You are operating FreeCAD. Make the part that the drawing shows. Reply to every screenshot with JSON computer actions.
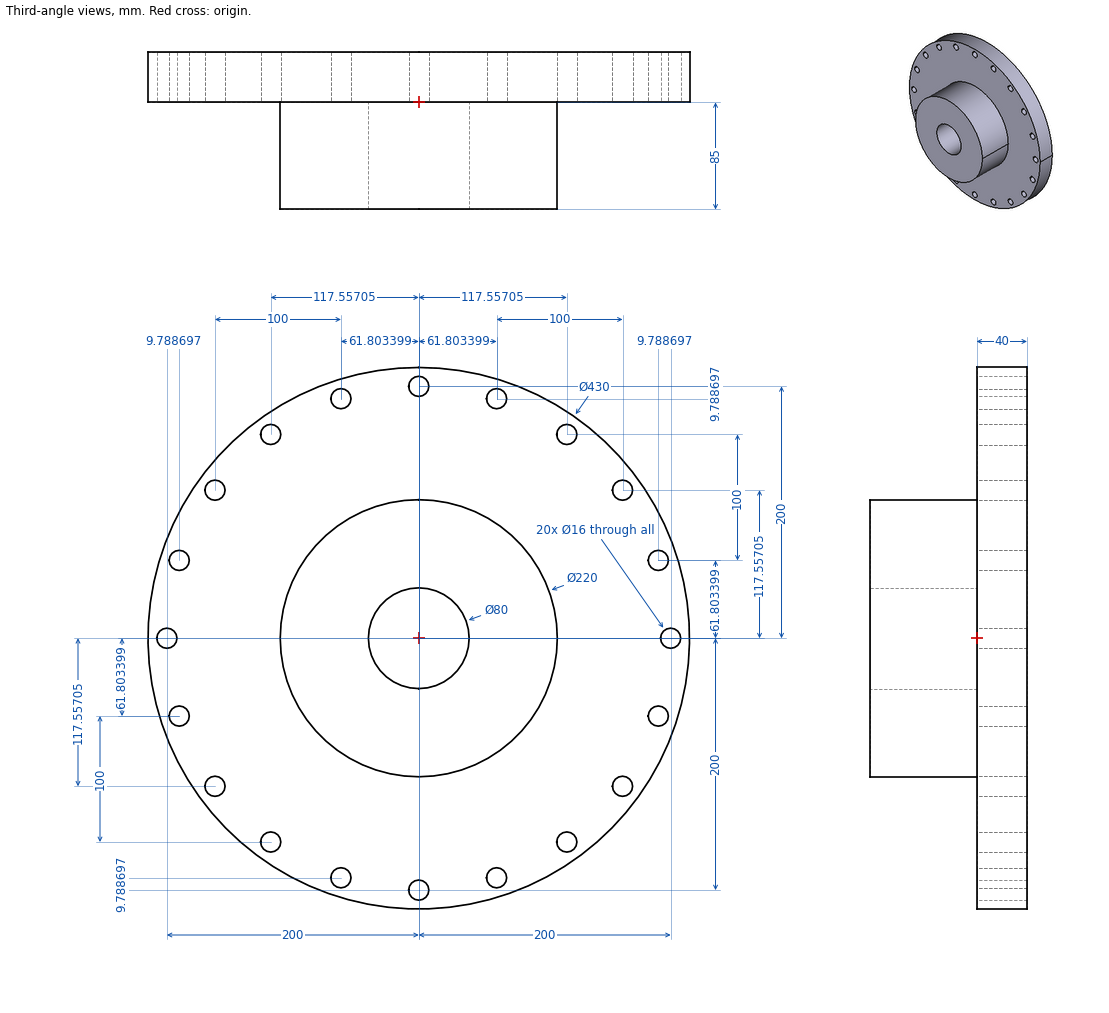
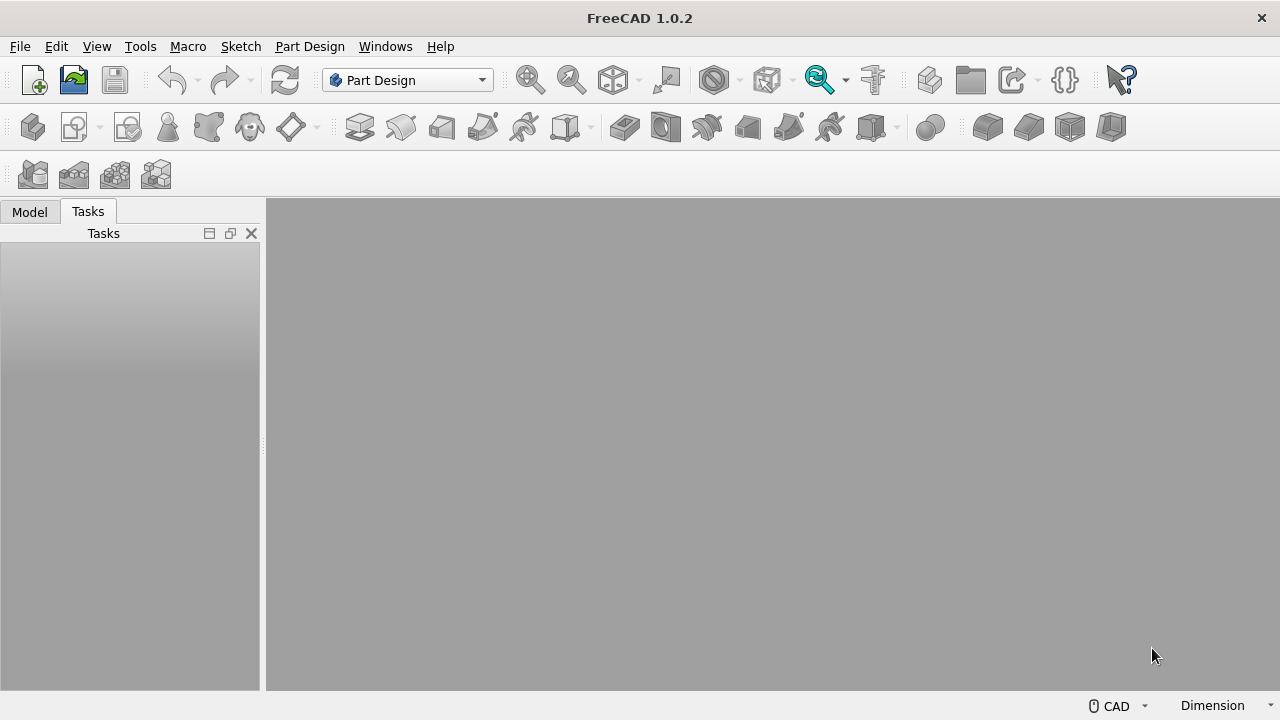
{"action": "key", "text": "ctrl+n"}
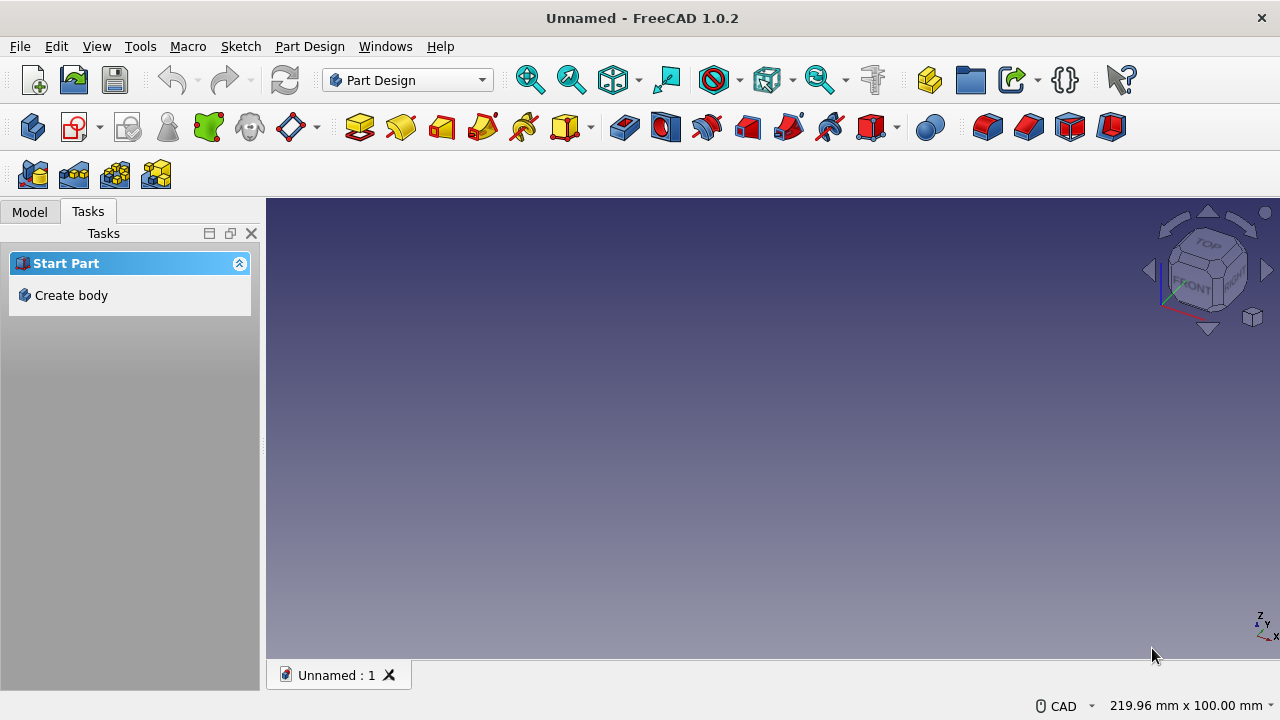
{"action": "left_click", "coordinate": [74, 128]}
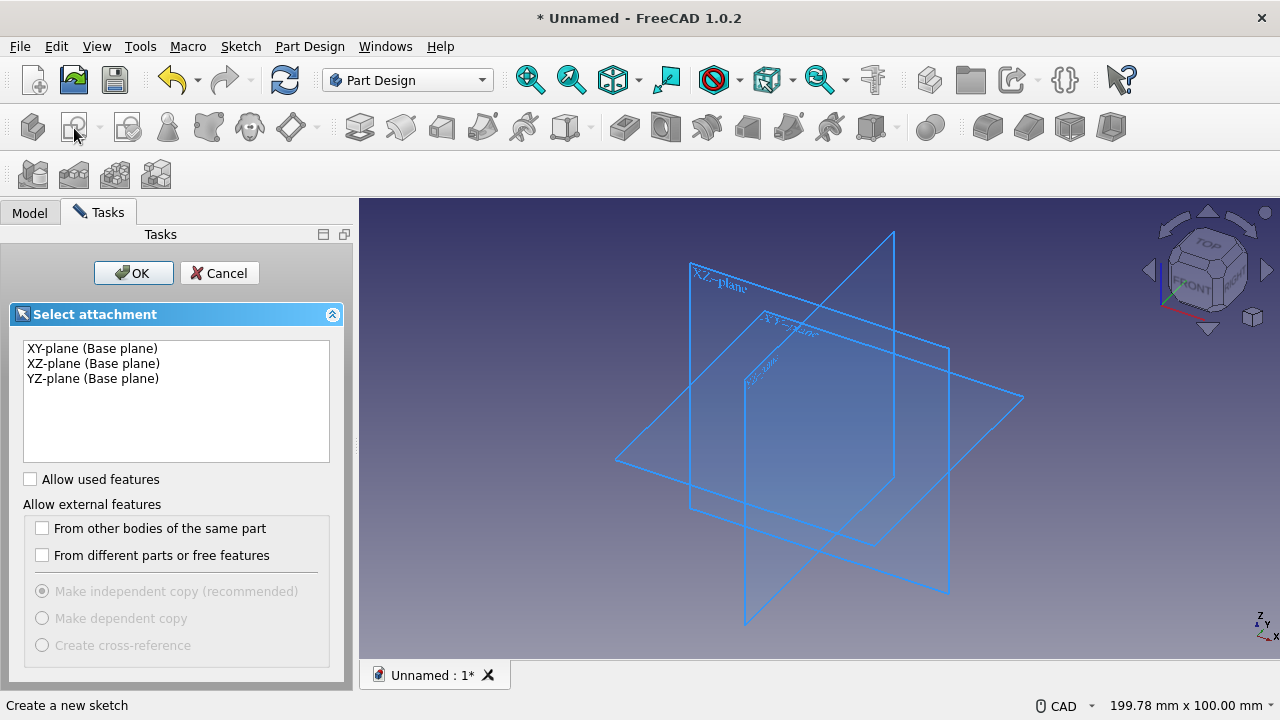
{"action": "left_click", "coordinate": [84, 364]}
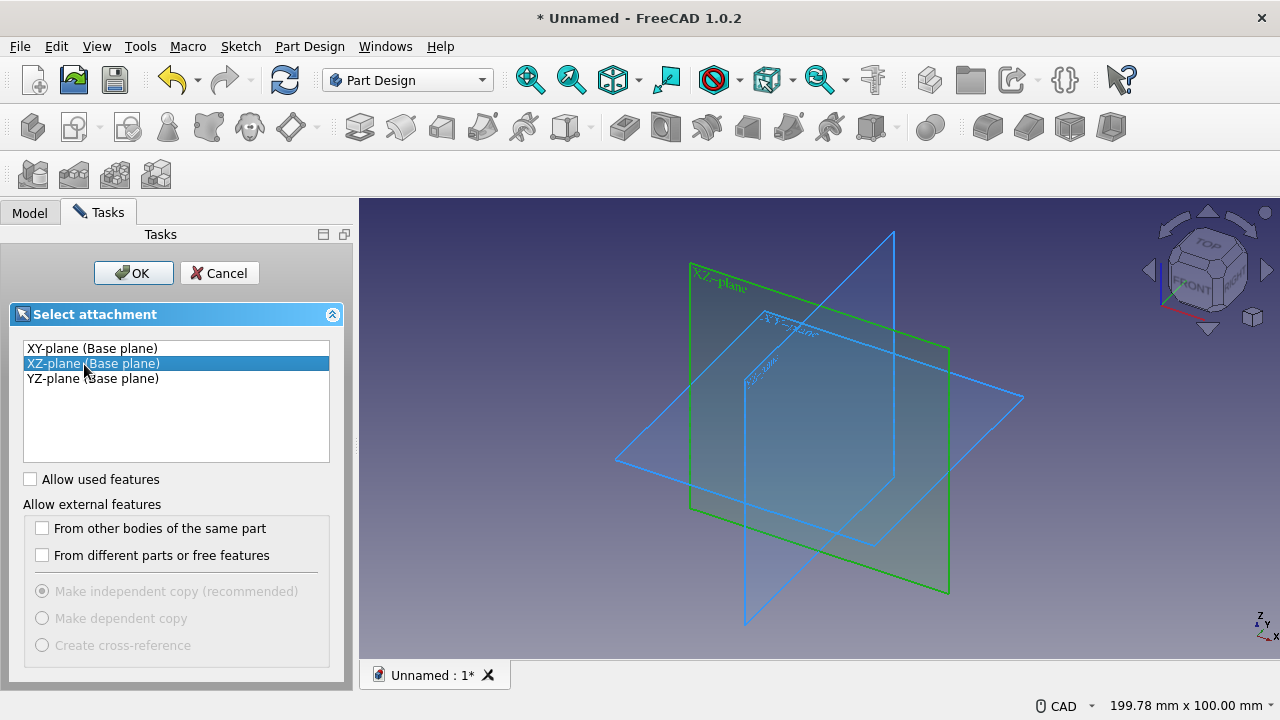
{"action": "left_click", "coordinate": [134, 273]}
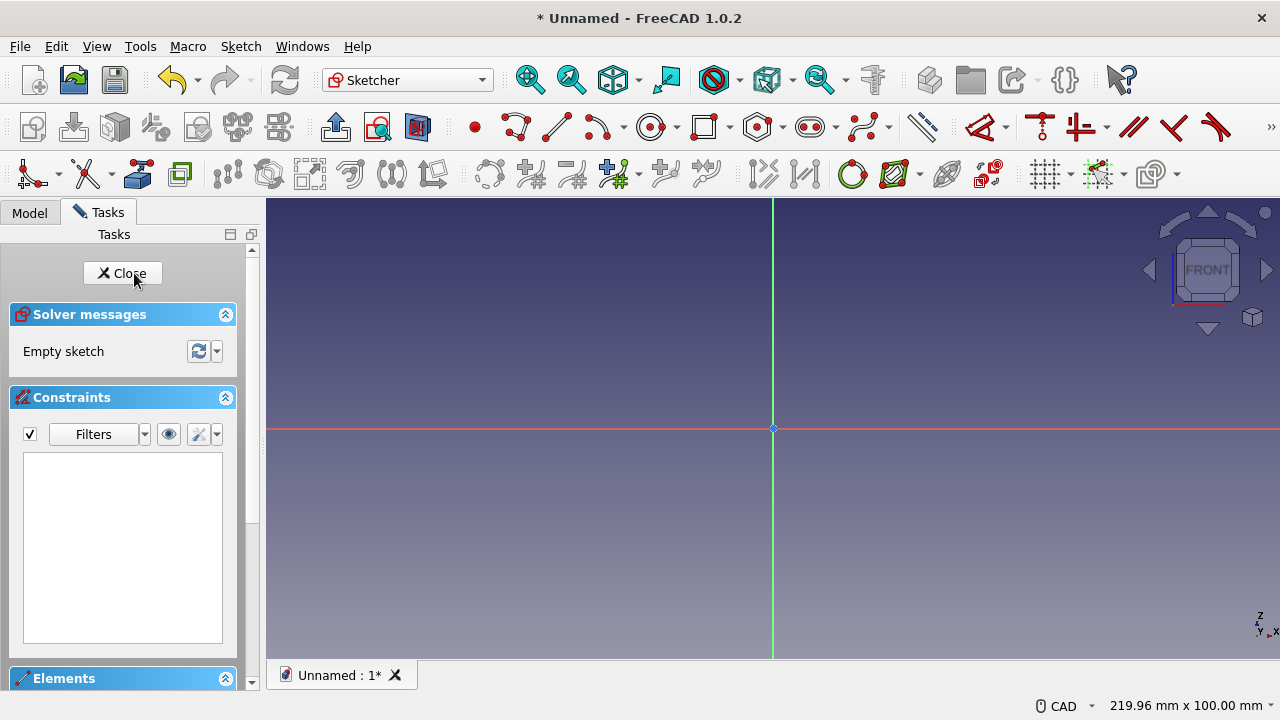
{"action": "scroll", "coordinate": [694, 428], "scroll_direction": "down", "scroll_amount": 10}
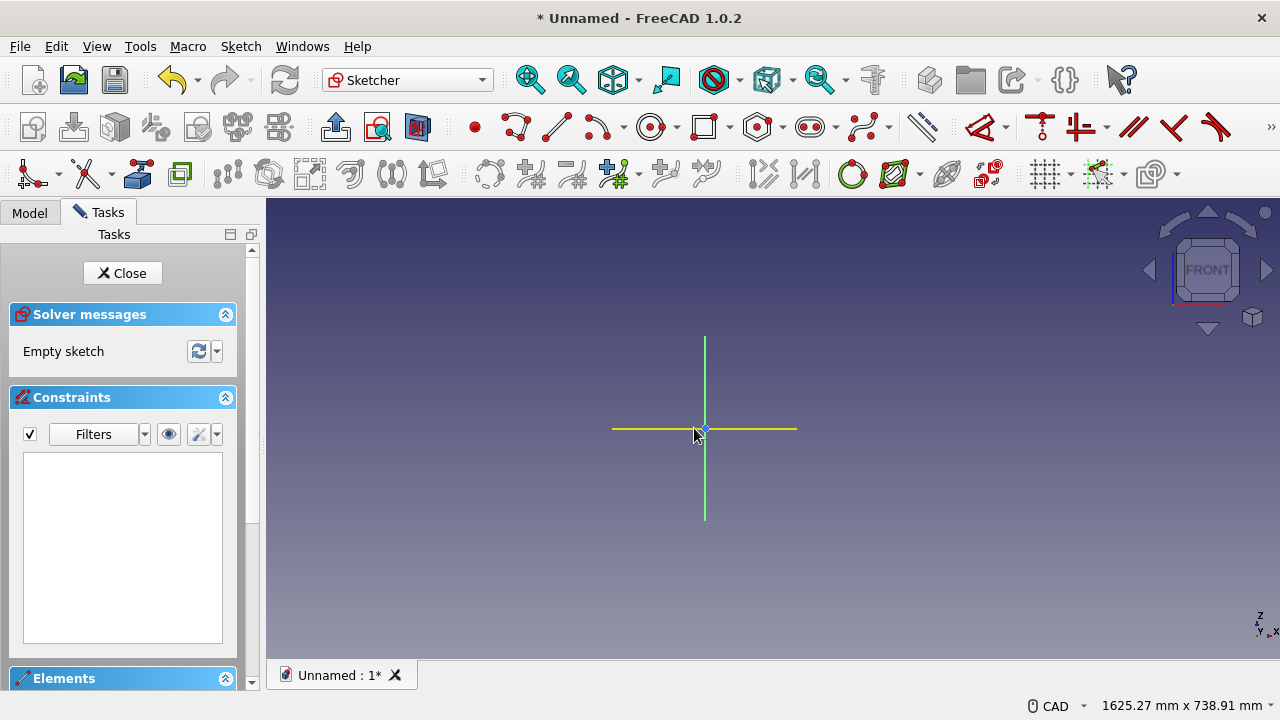
{"action": "left_click", "coordinate": [650, 128]}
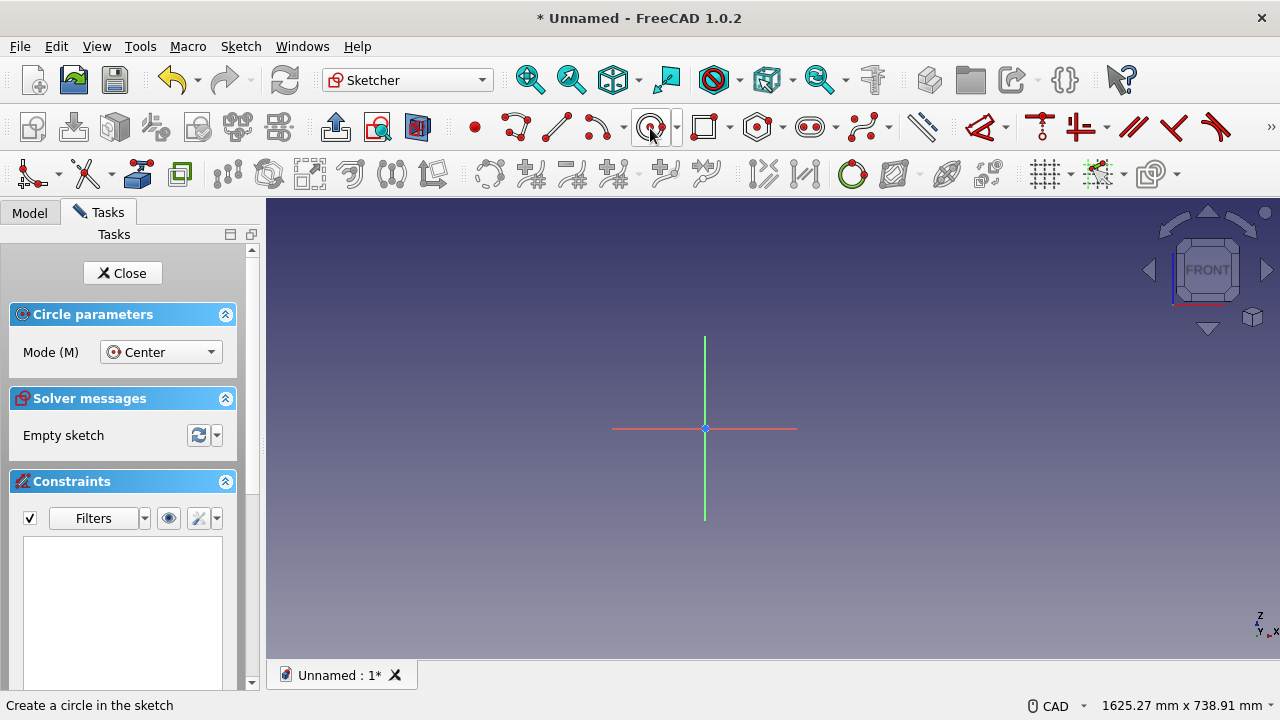
{"action": "left_click", "coordinate": [705, 428]}
{"action": "left_click", "coordinate": [800, 334]}
{"action": "key", "text": "Escape"}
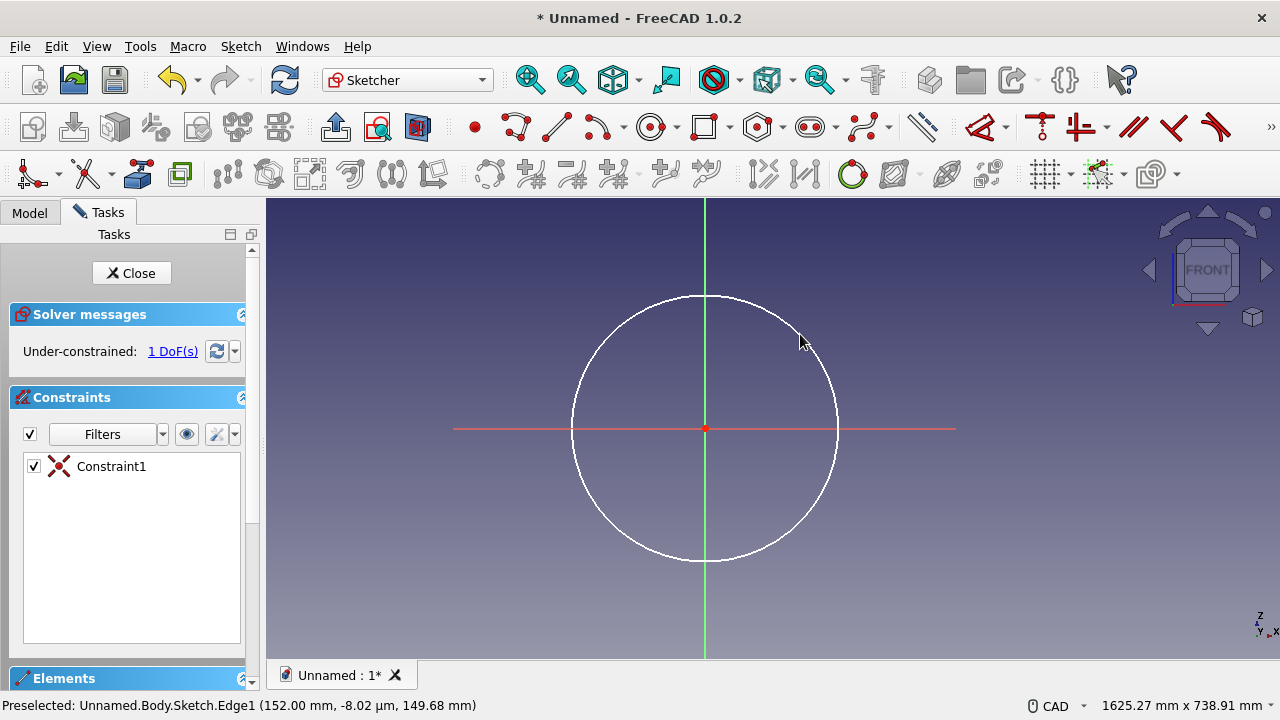
{"action": "left_click", "coordinate": [980, 128]}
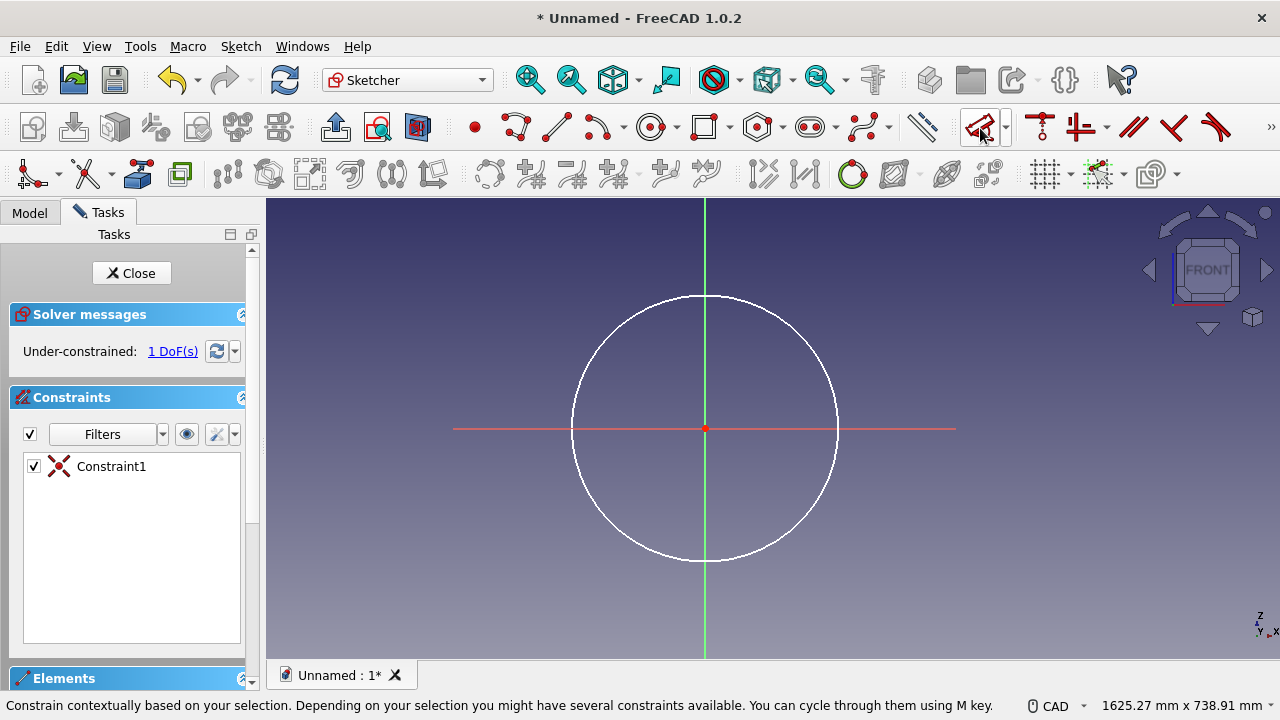
{"action": "left_click", "coordinate": [799, 334]}
{"action": "left_click", "coordinate": [822, 311]}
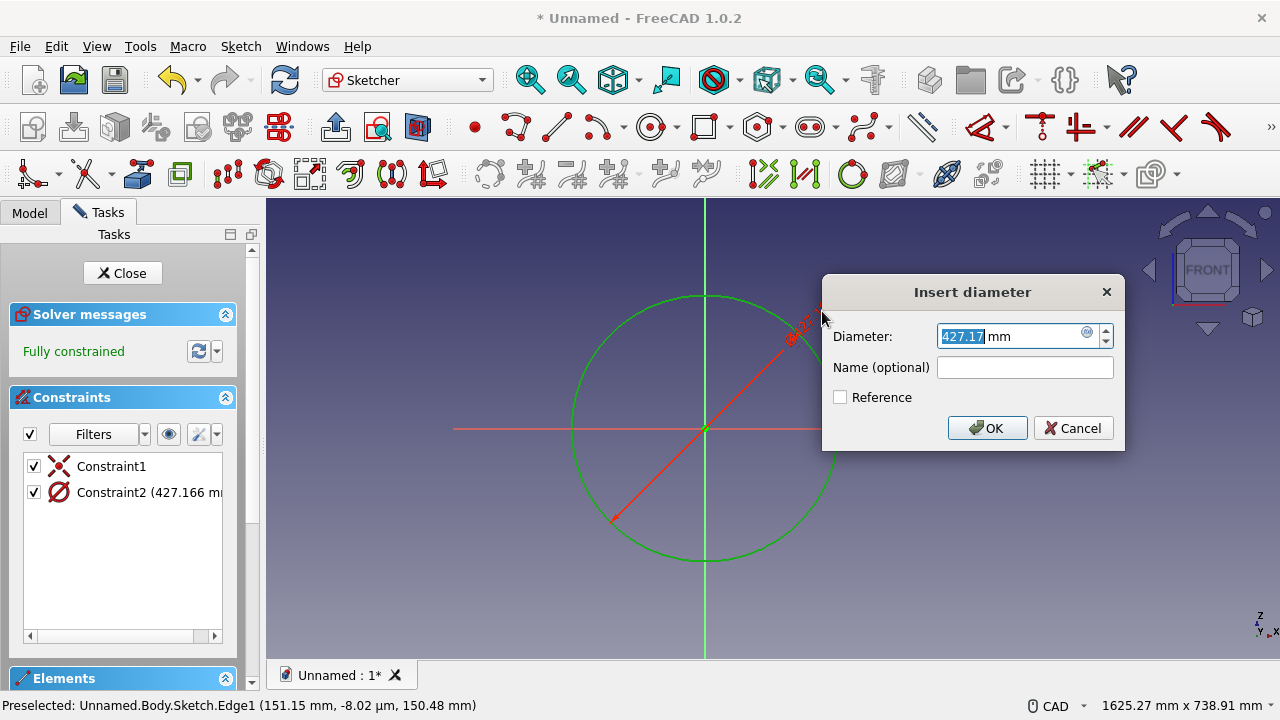
{"action": "type", "text": "430"}
{"action": "key", "text": "Return"}
{"action": "key", "text": "Escape"}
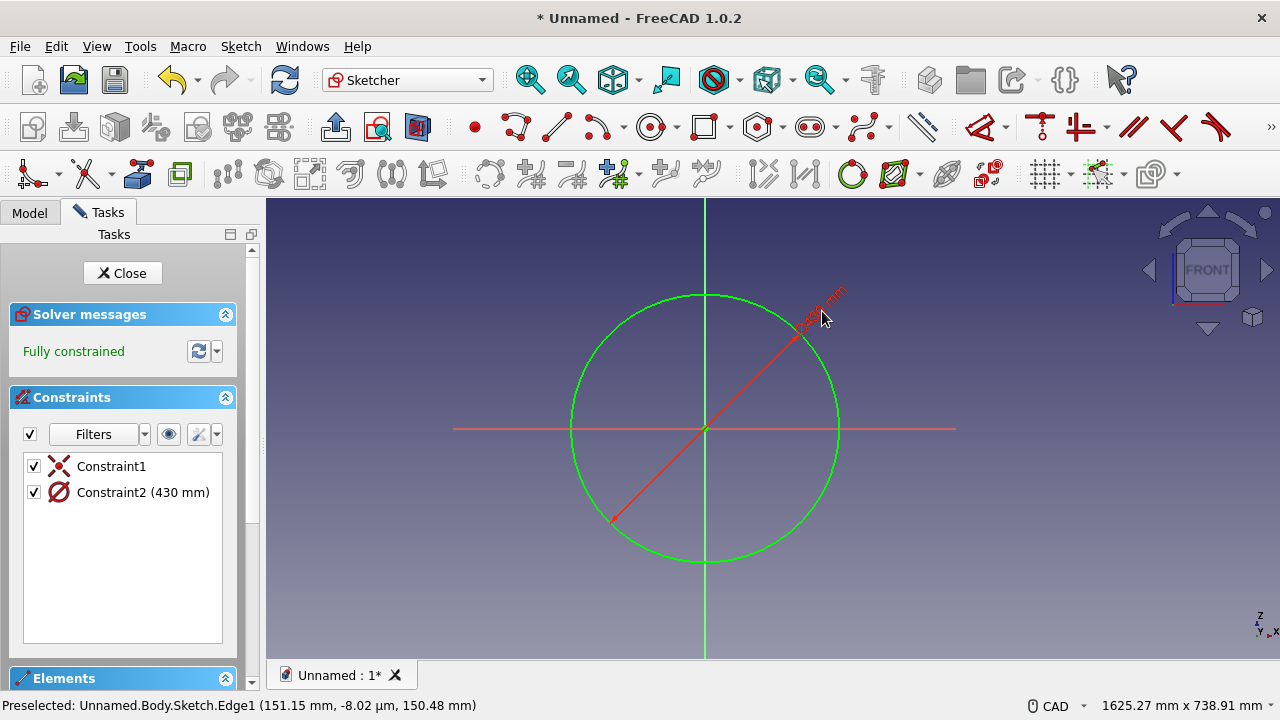
{"action": "left_click", "coordinate": [123, 273]}